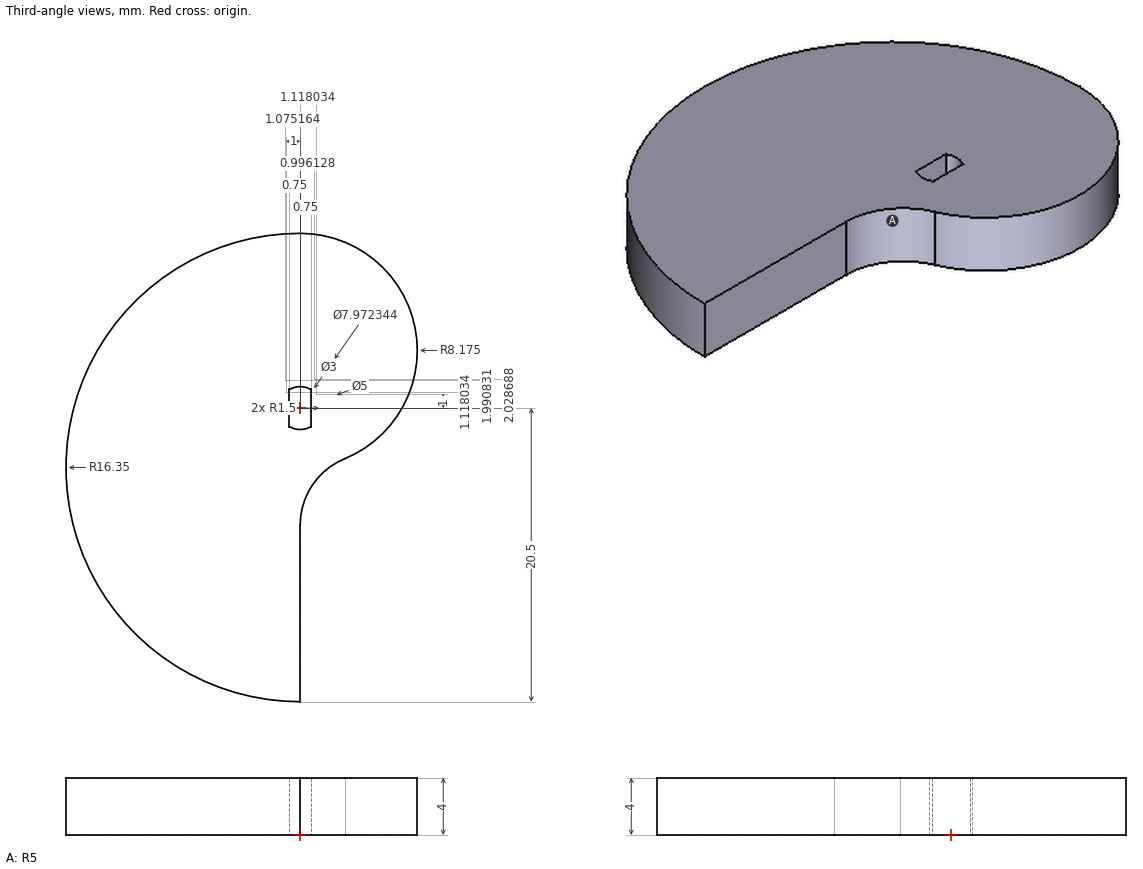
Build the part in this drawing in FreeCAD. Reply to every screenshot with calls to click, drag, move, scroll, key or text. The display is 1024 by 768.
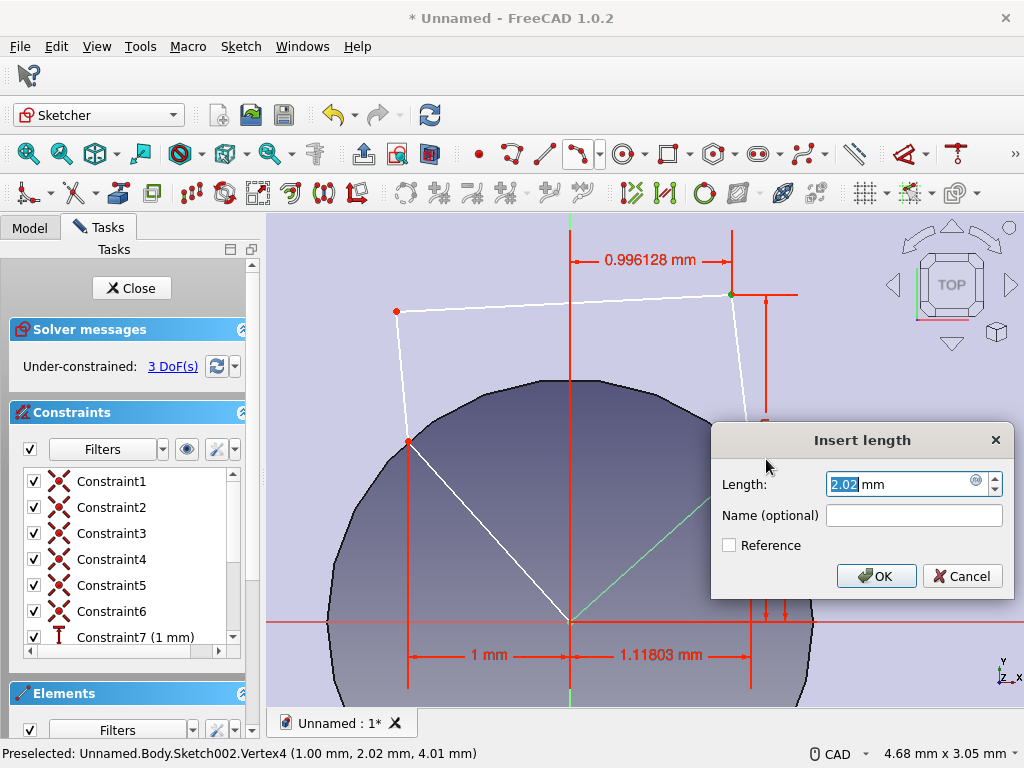
text(2.028688)
key(Return)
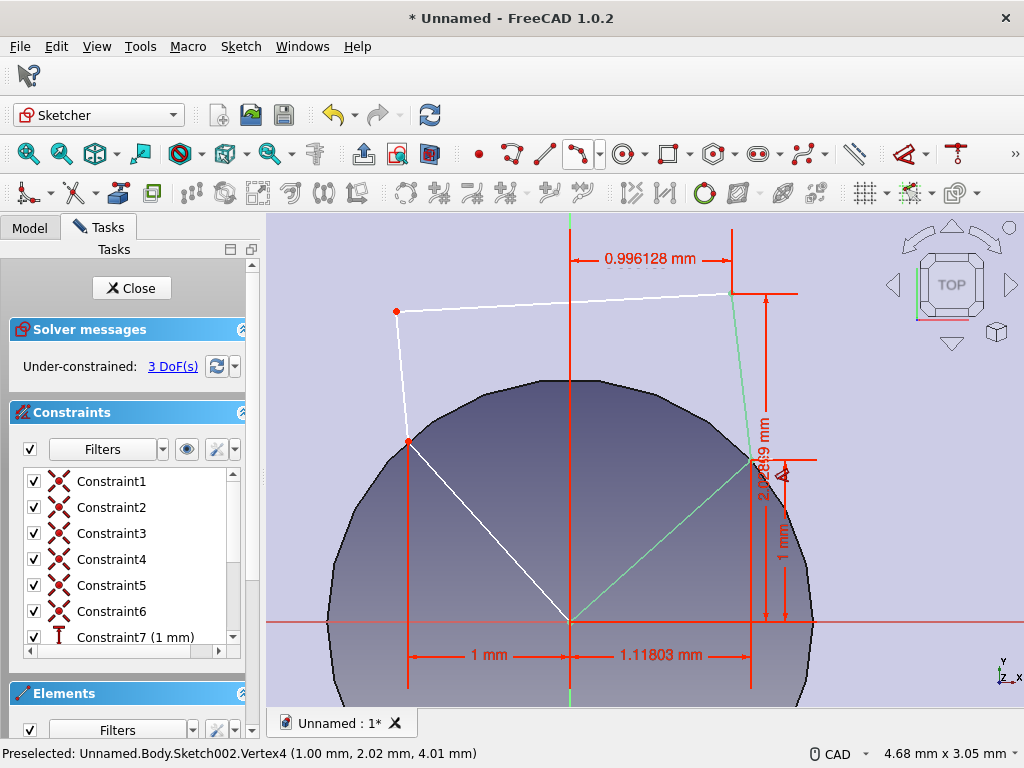
click(396, 312)
click(483, 278)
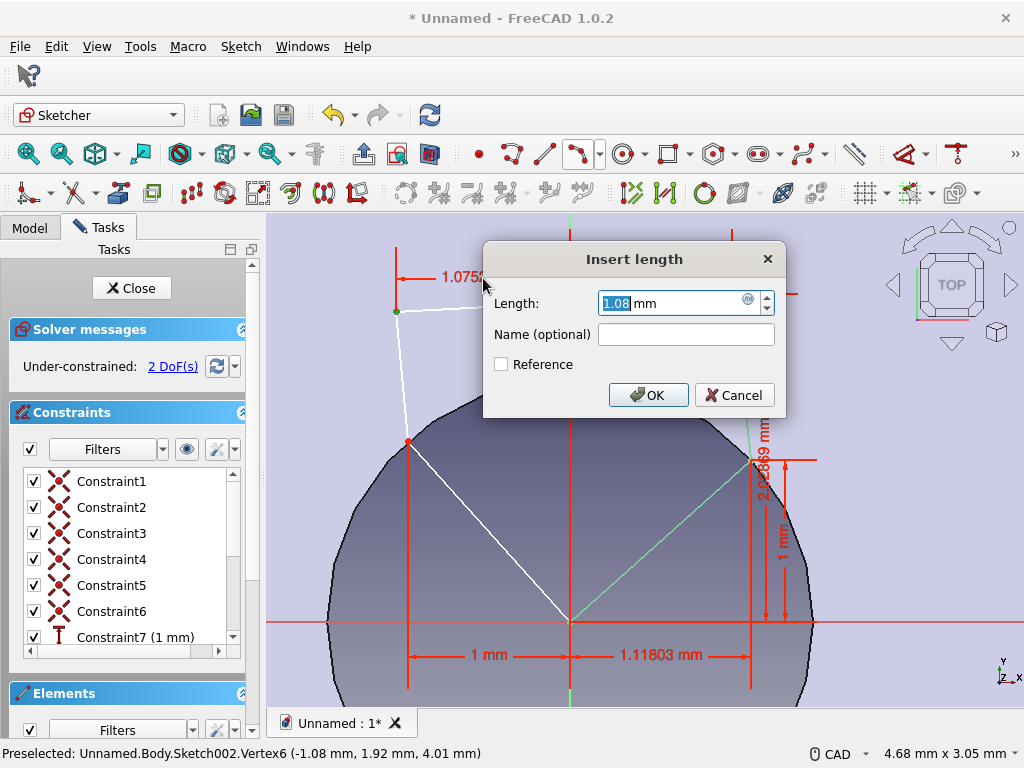
text(1.075164)
key(Return)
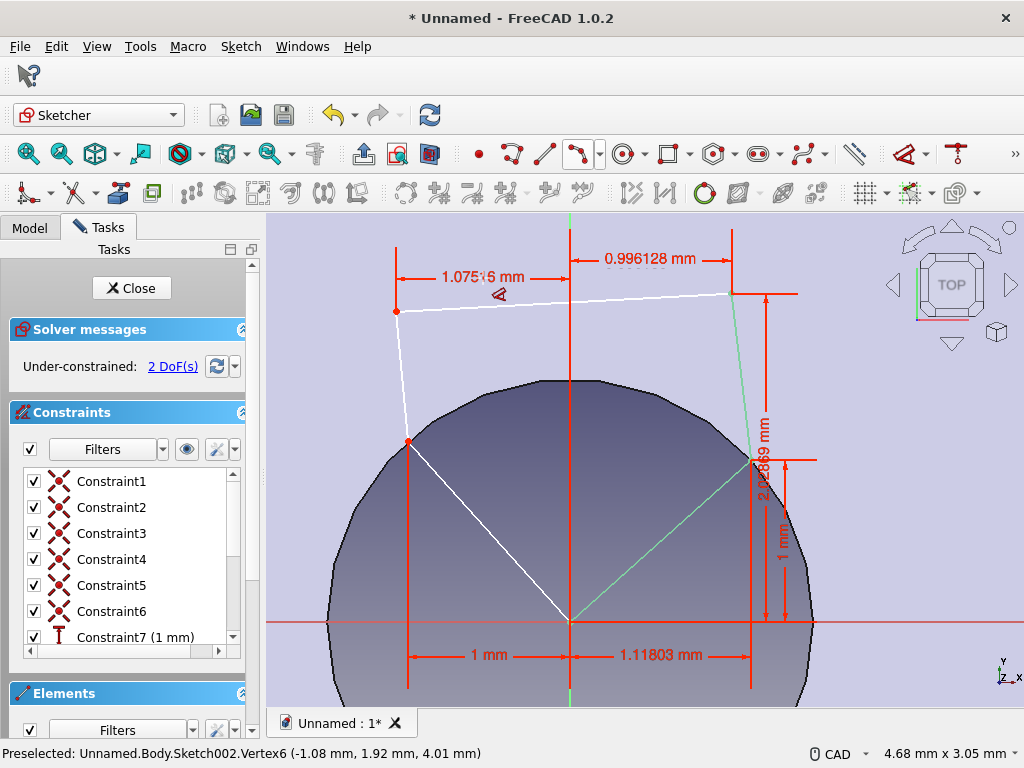
click(396, 312)
click(362, 467)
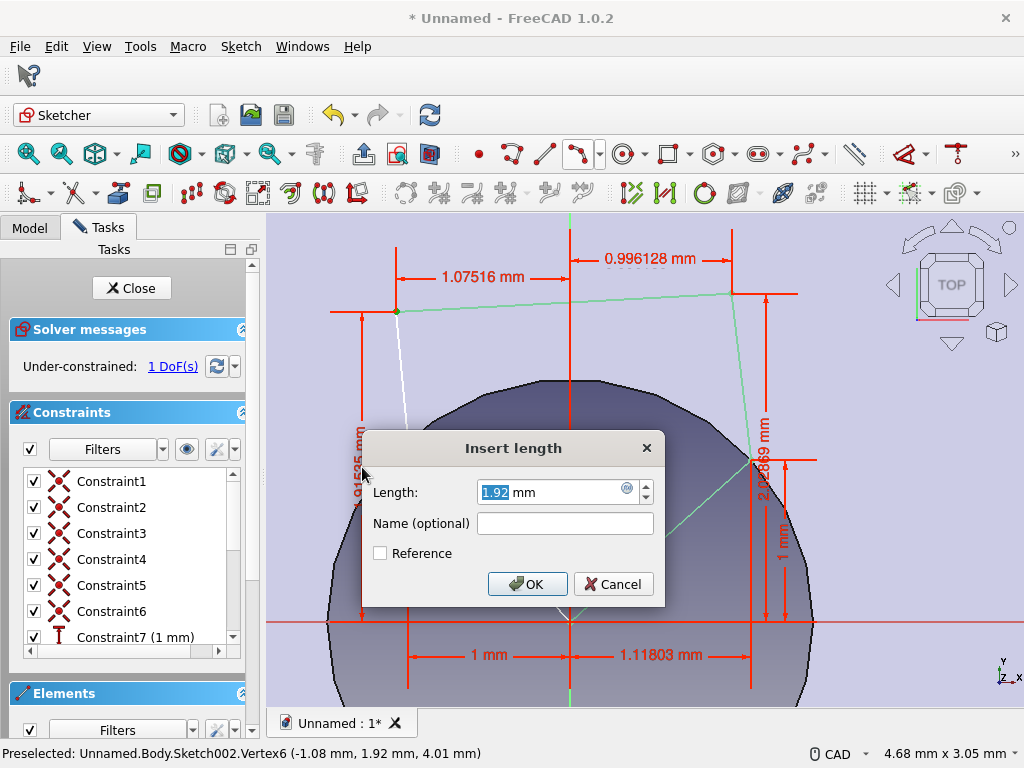
text(1.990831)
key(Return)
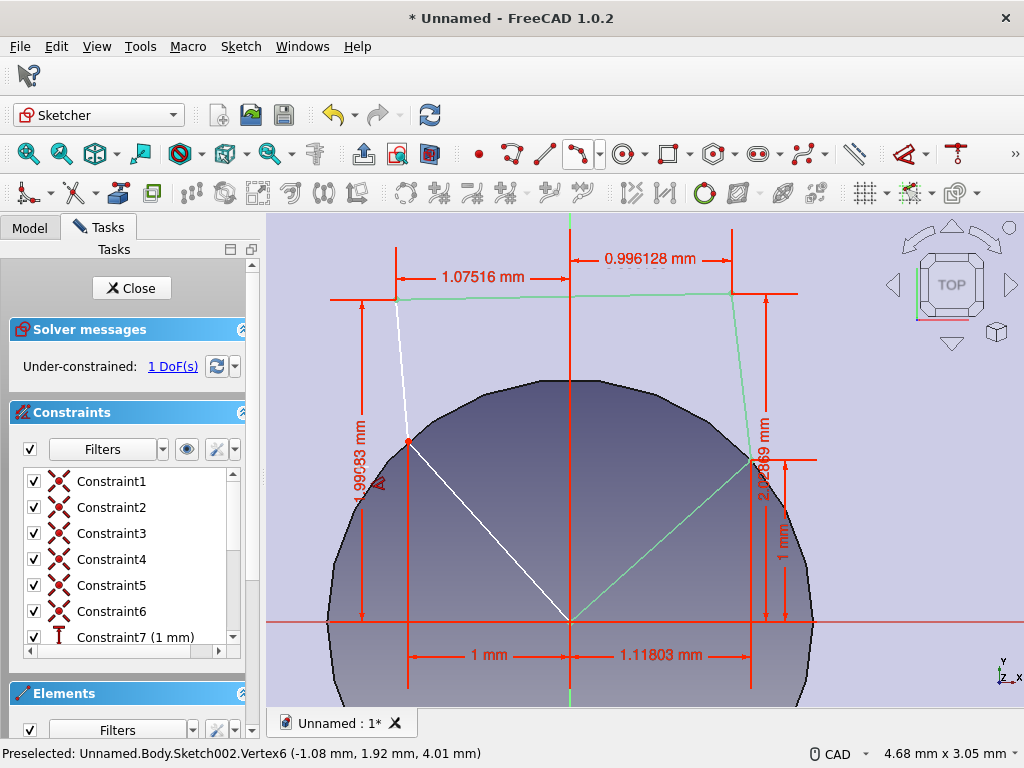
click(408, 442)
click(374, 532)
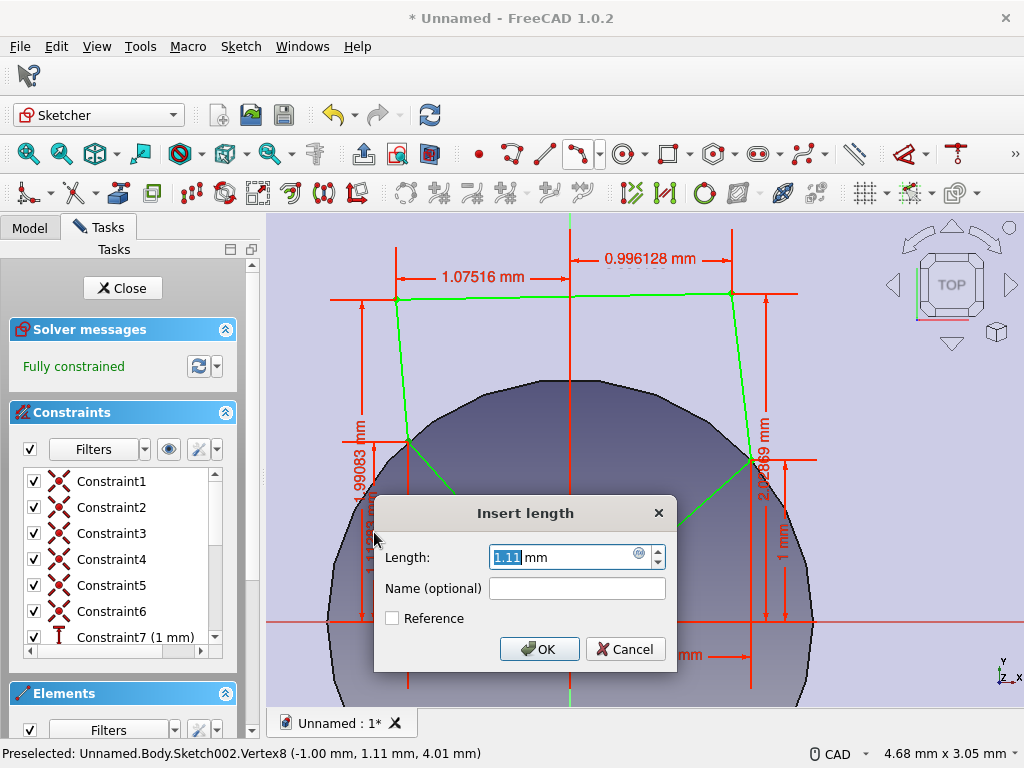
text(1.118034)
key(Return)
key(Escape)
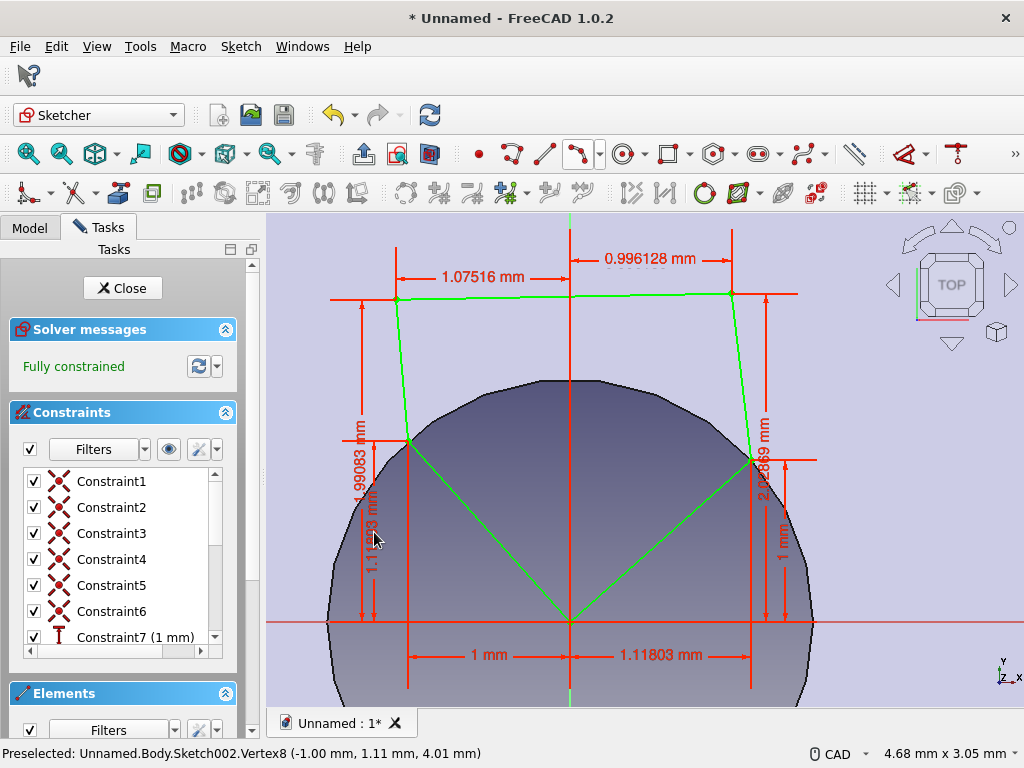
click(123, 288)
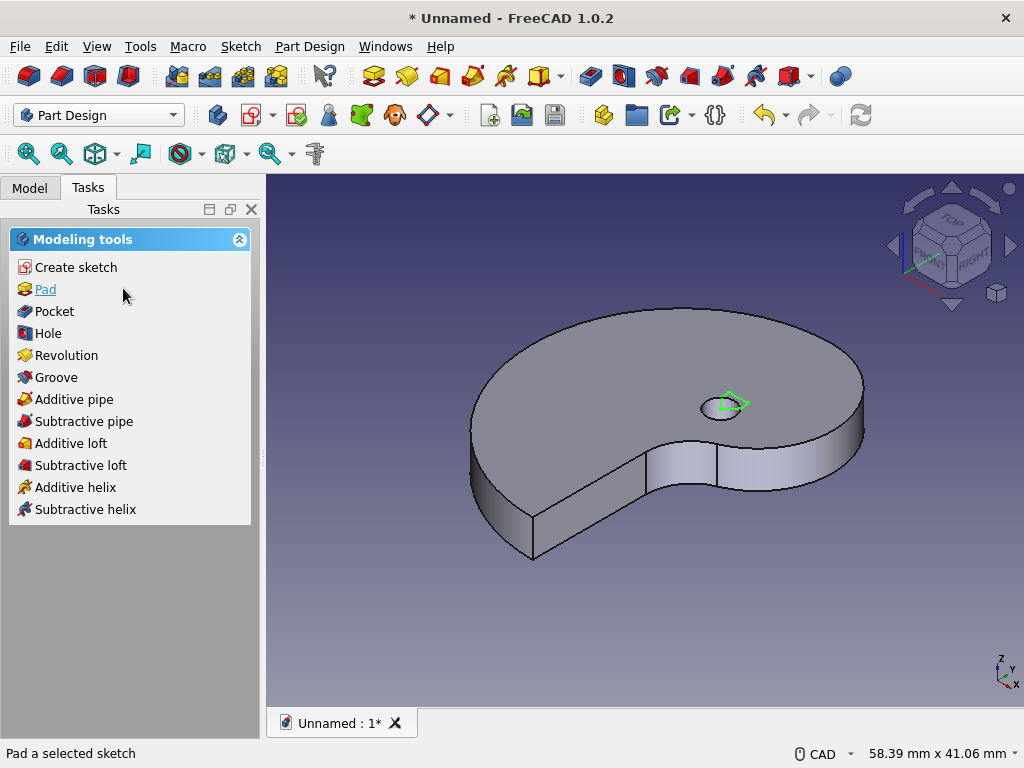
click(374, 76)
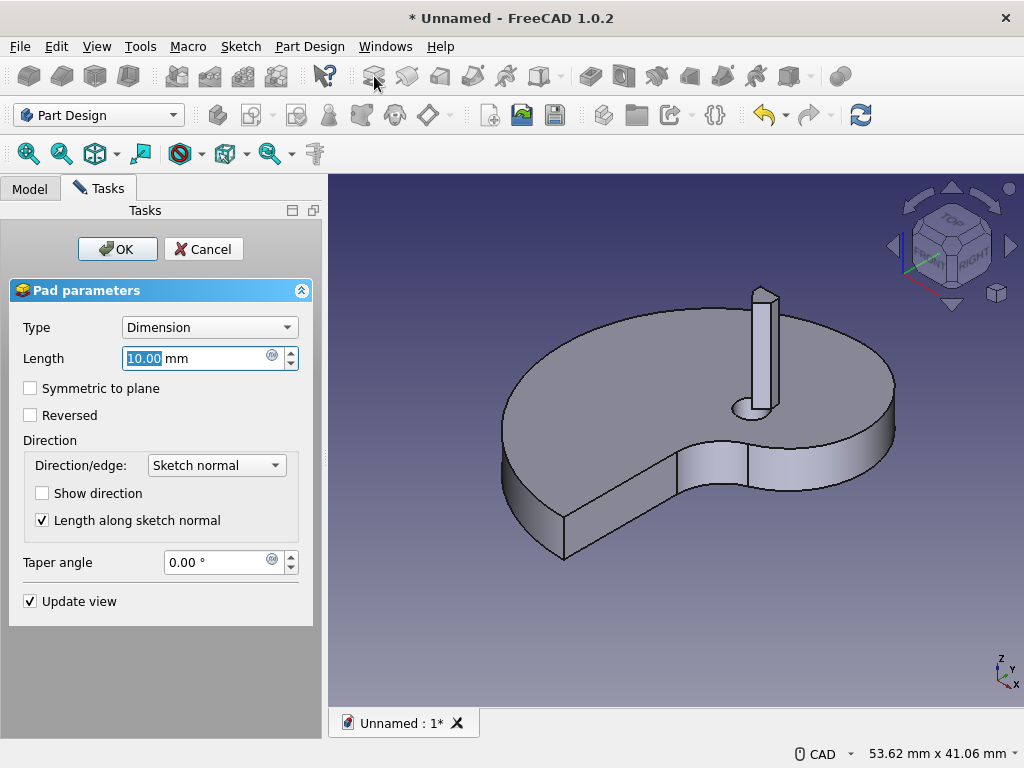
text(4)
key(Tab)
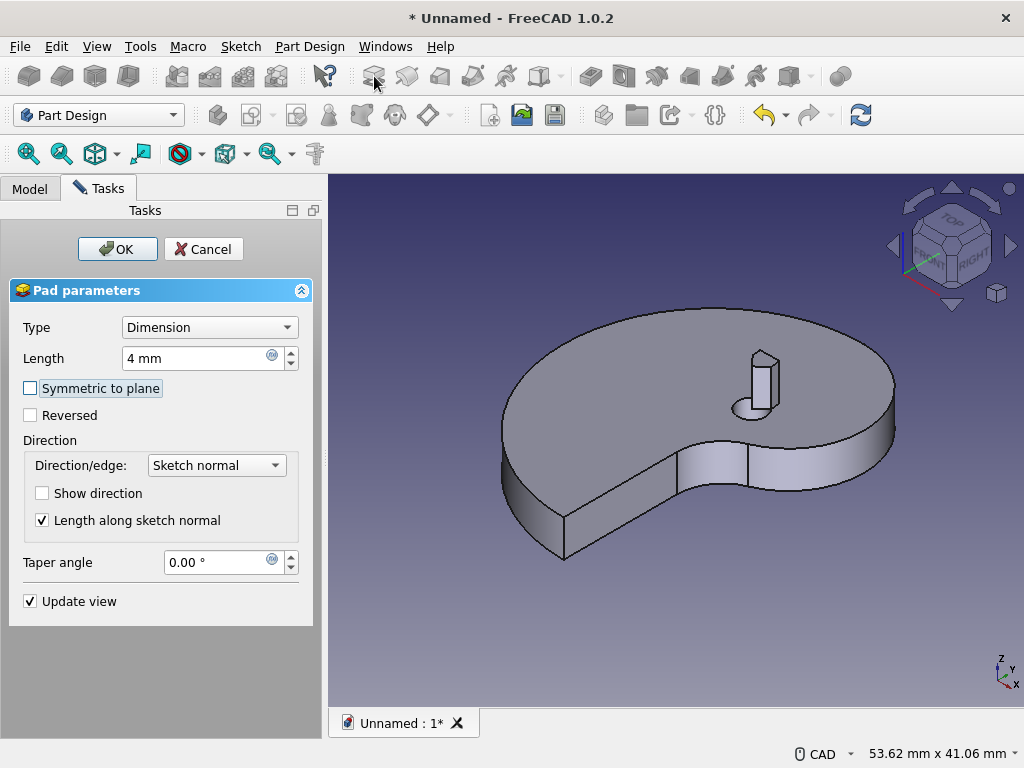
click(31, 415)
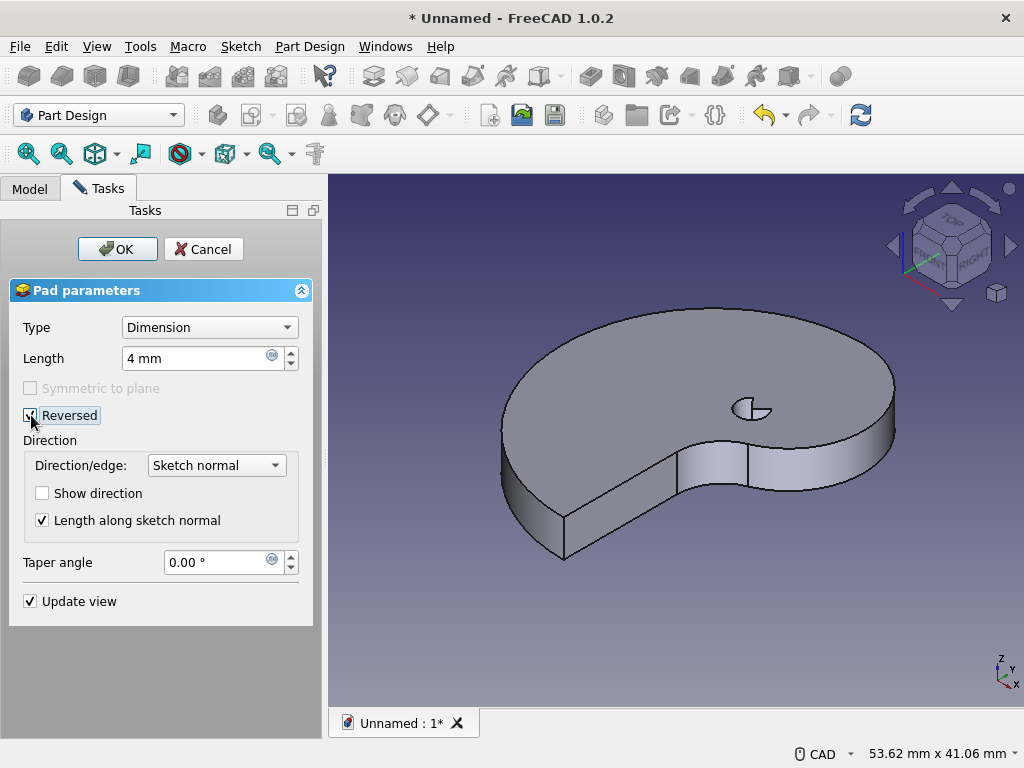
click(118, 249)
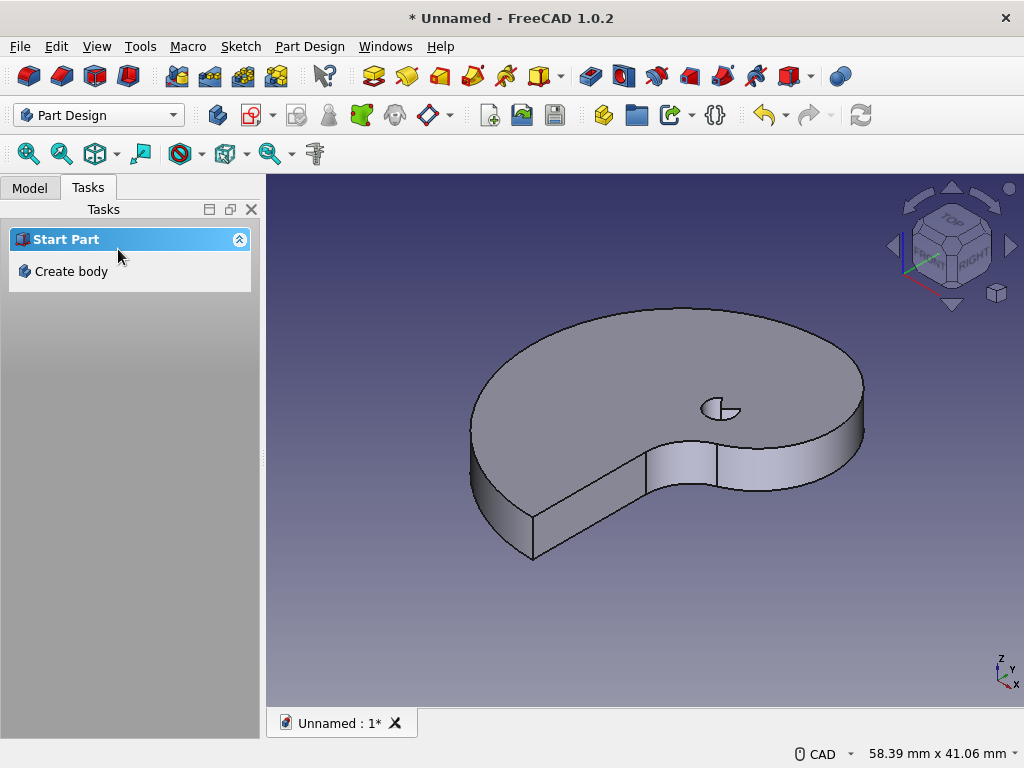
click(570, 414)